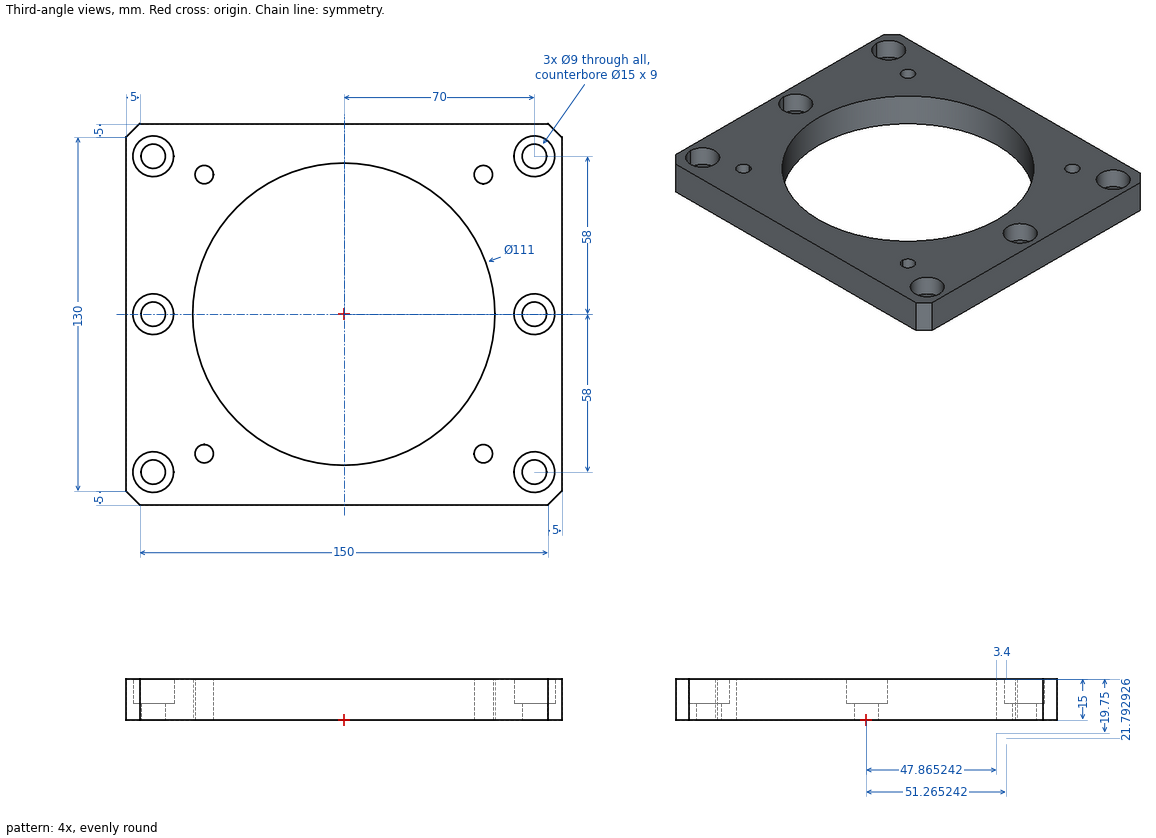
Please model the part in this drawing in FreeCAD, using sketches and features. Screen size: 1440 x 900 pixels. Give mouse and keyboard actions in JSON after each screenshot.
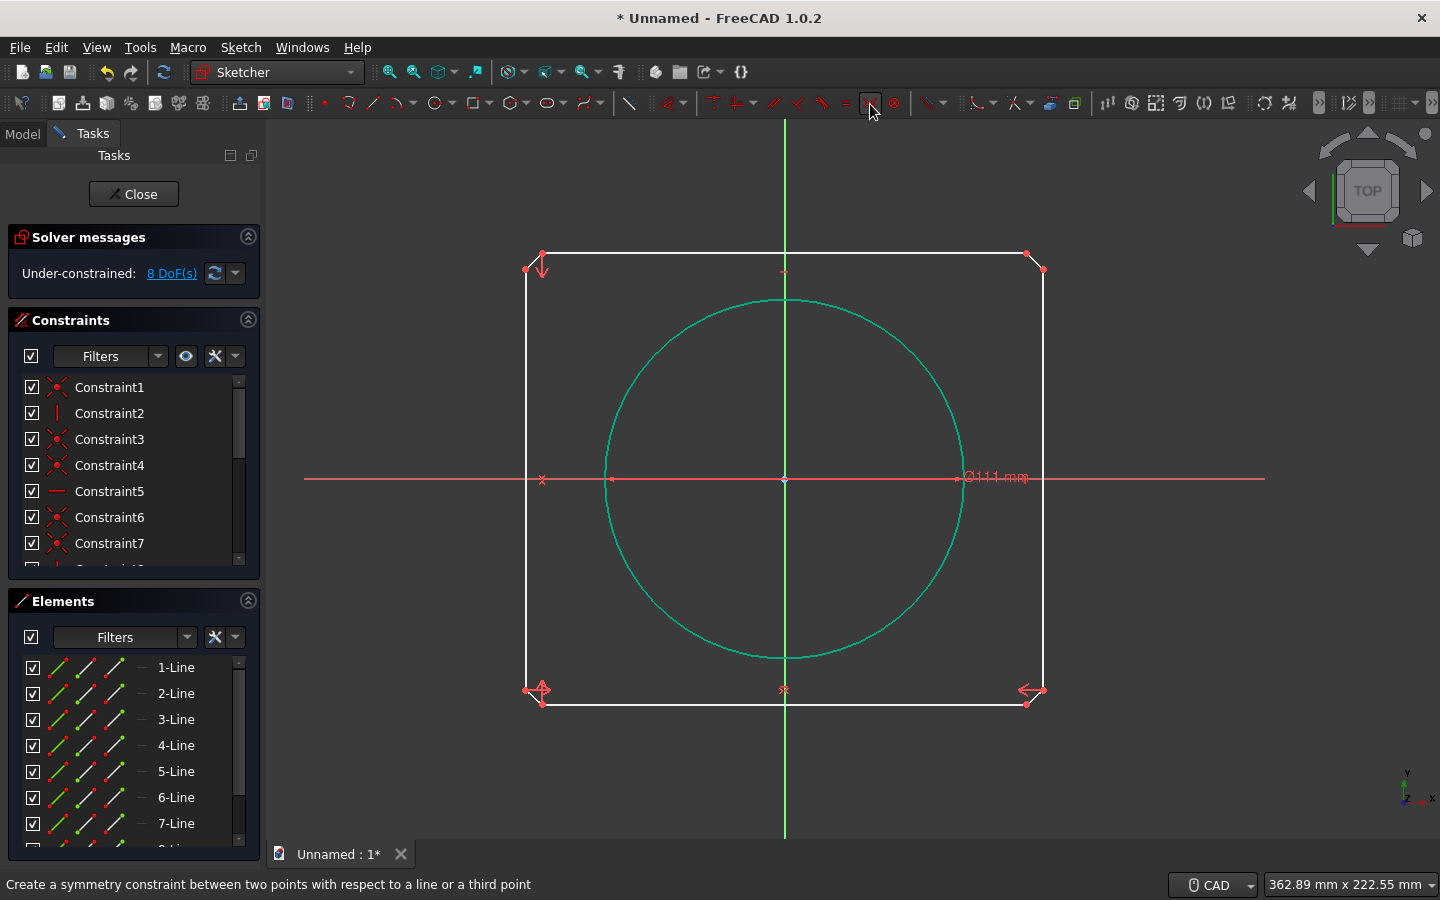
{"action": "scroll", "coordinate": [536, 260], "scroll_direction": "up", "scroll_amount": 5}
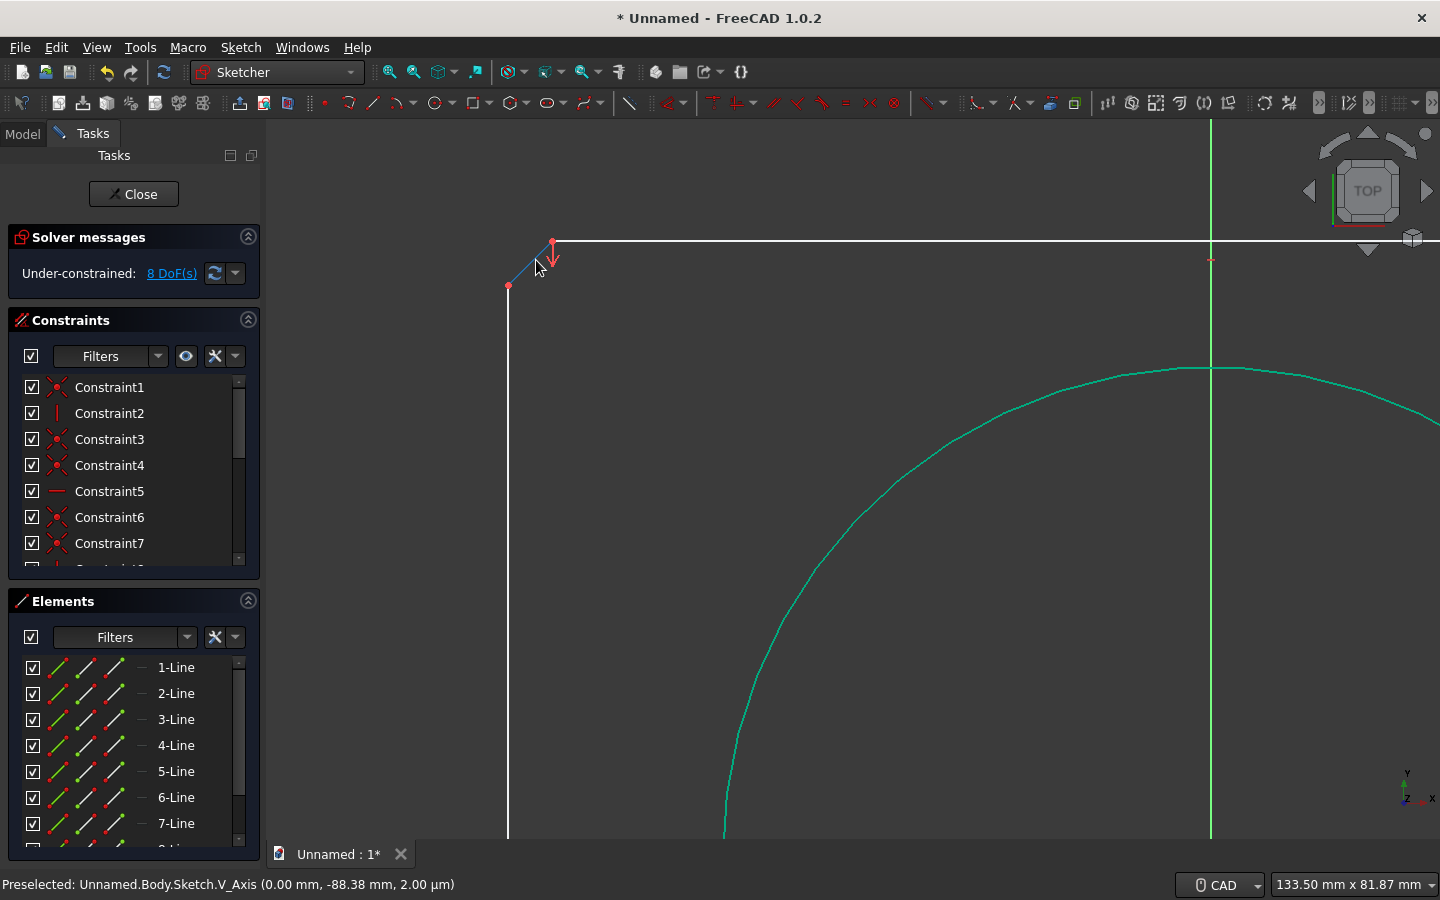
{"action": "left_click", "coordinate": [535, 259]}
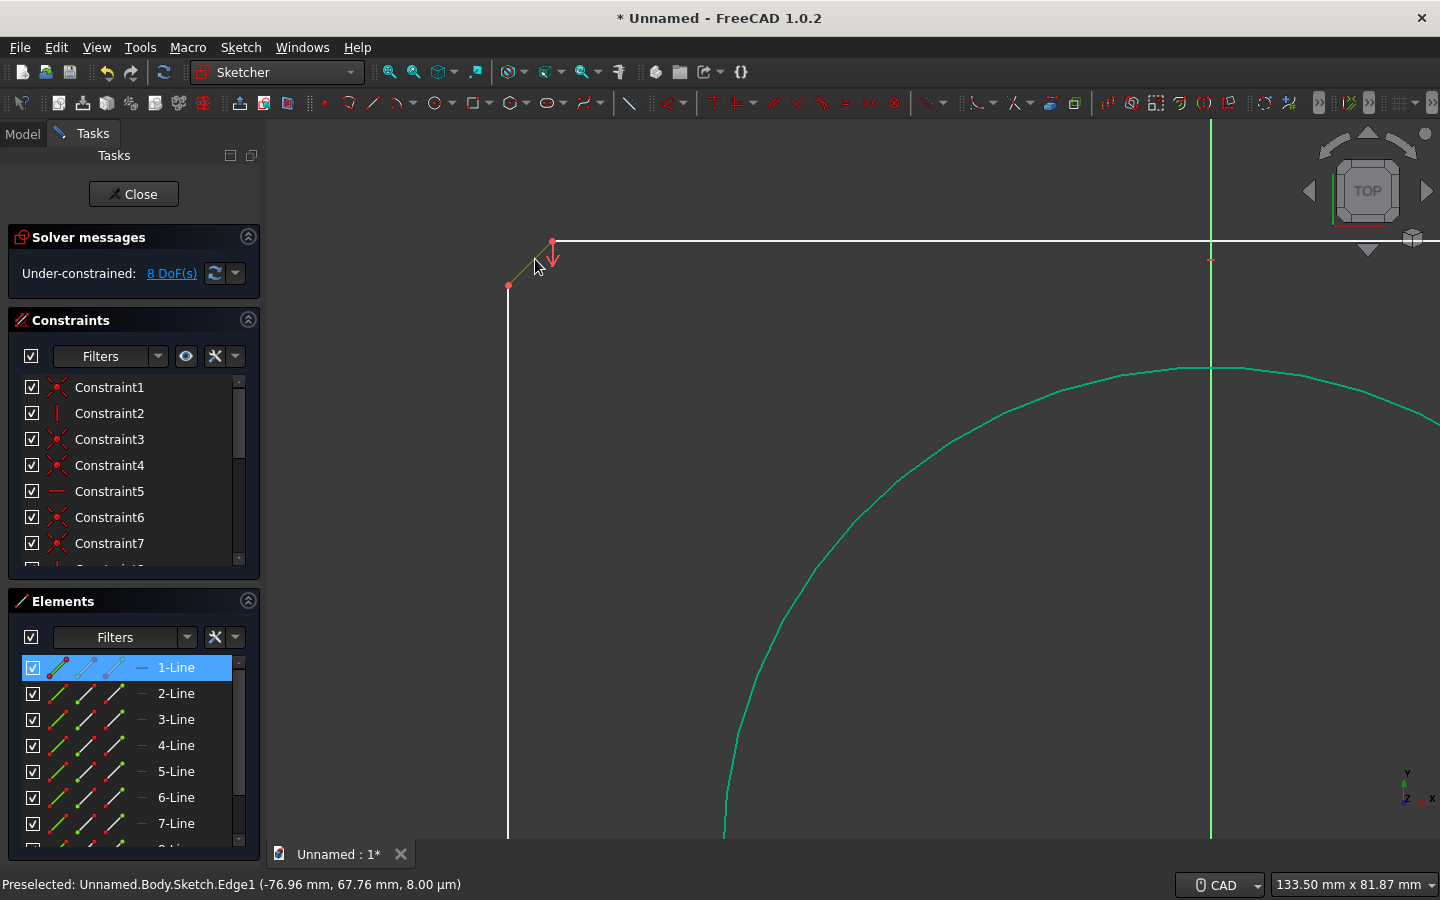
{"action": "key", "text": "l"}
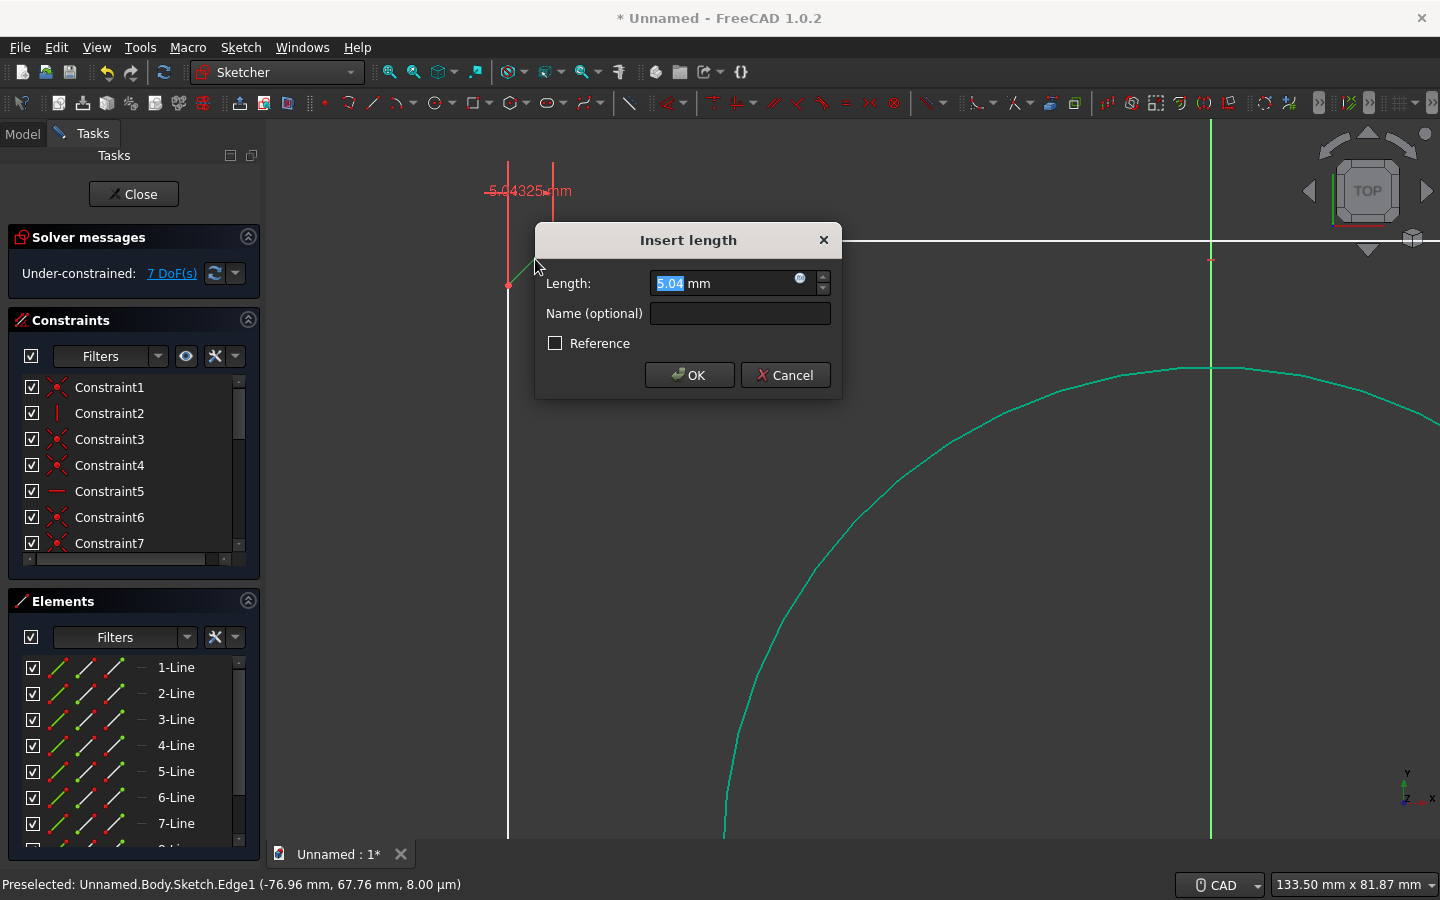
{"action": "type", "text": "5"}
{"action": "key", "text": "Return"}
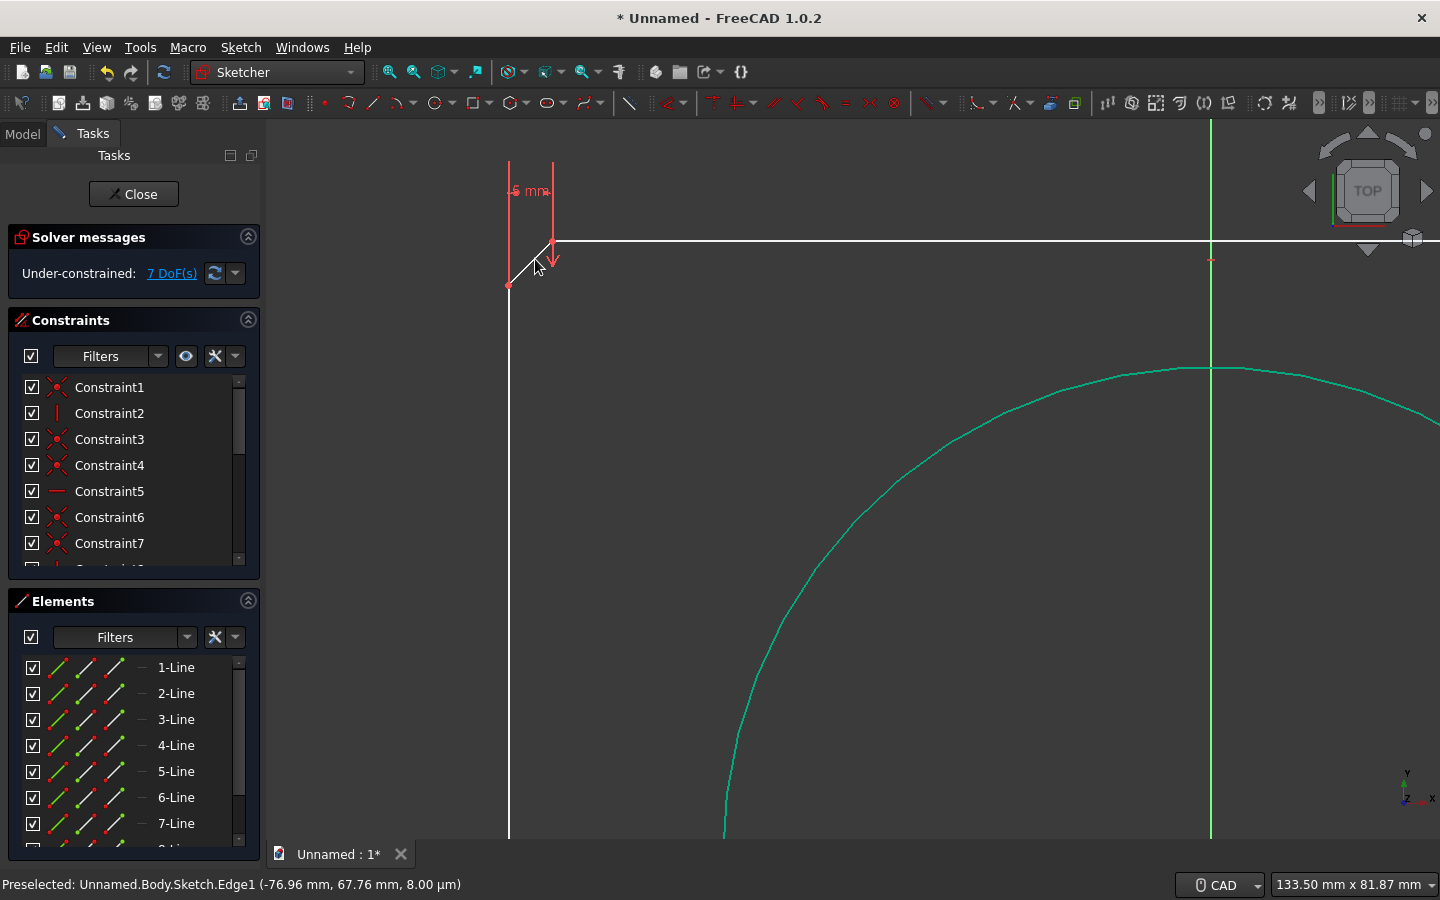
{"action": "left_click", "coordinate": [539, 254]}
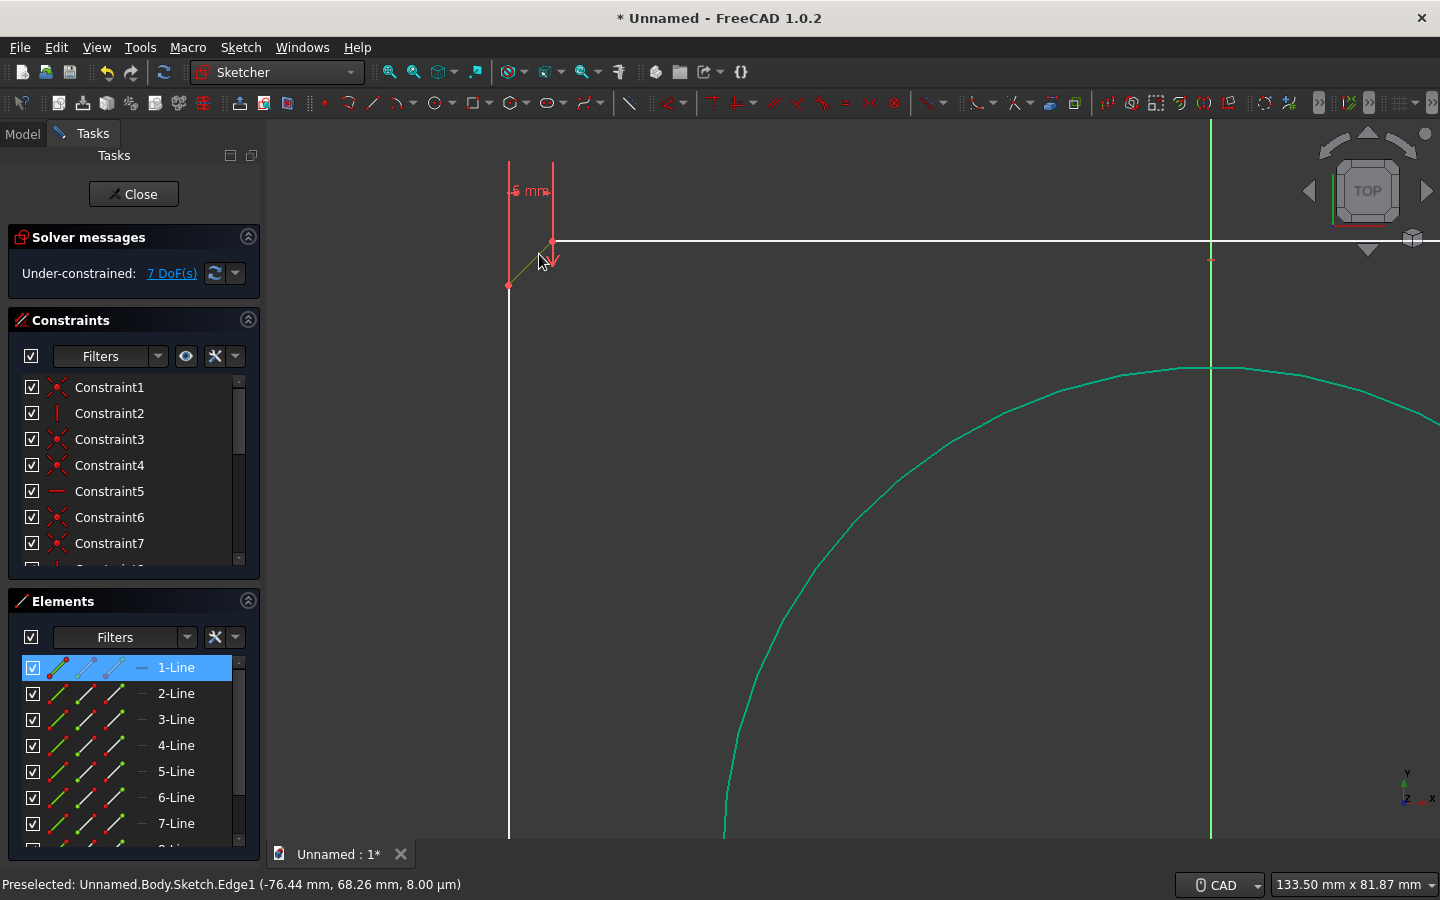
{"action": "key", "text": "i"}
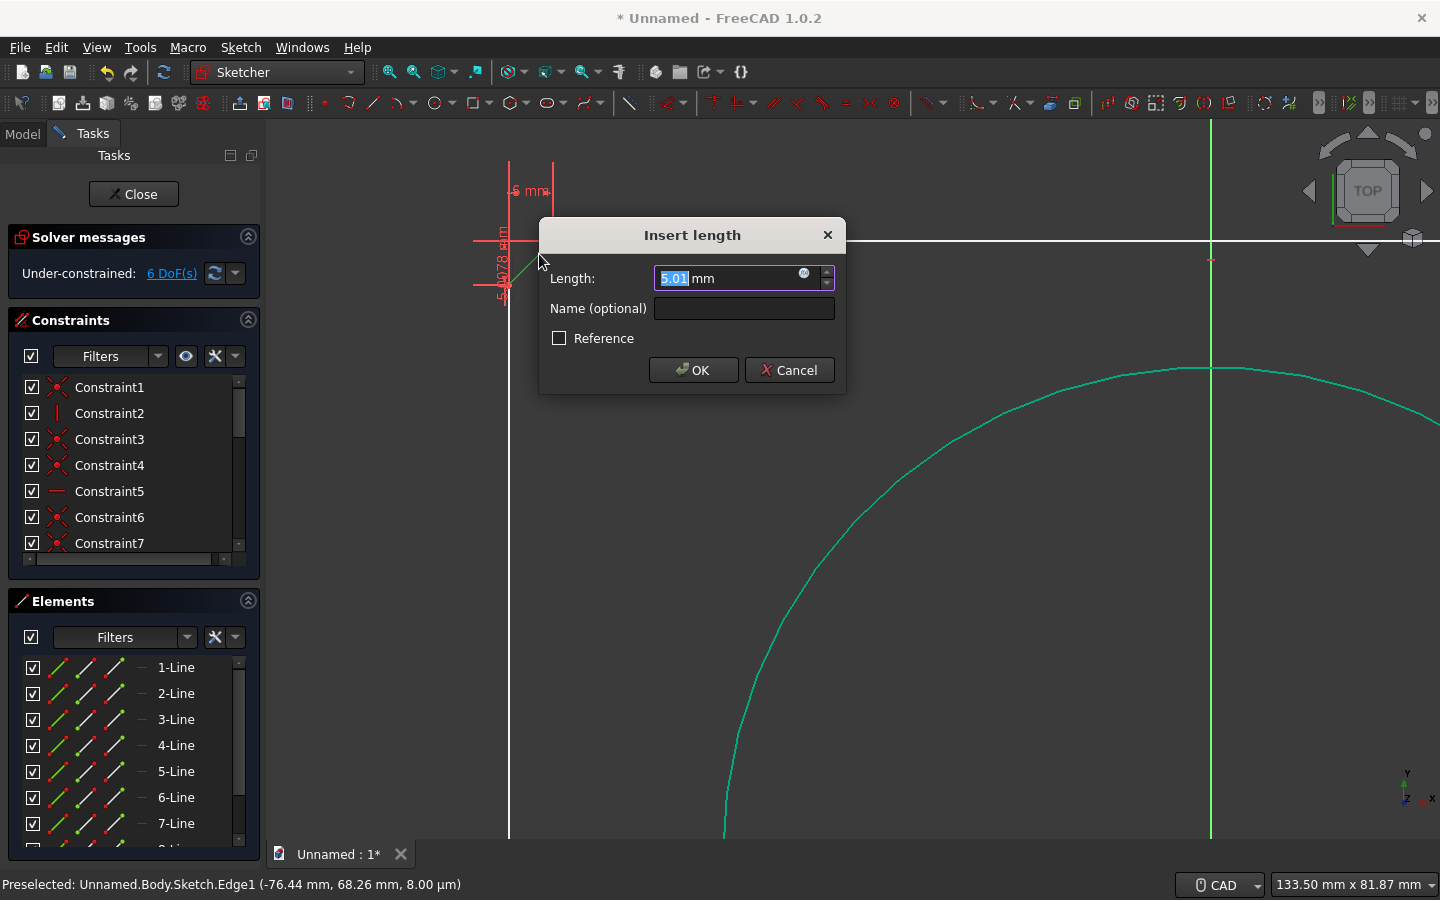
{"action": "type", "text": "5"}
{"action": "key", "text": "Return"}